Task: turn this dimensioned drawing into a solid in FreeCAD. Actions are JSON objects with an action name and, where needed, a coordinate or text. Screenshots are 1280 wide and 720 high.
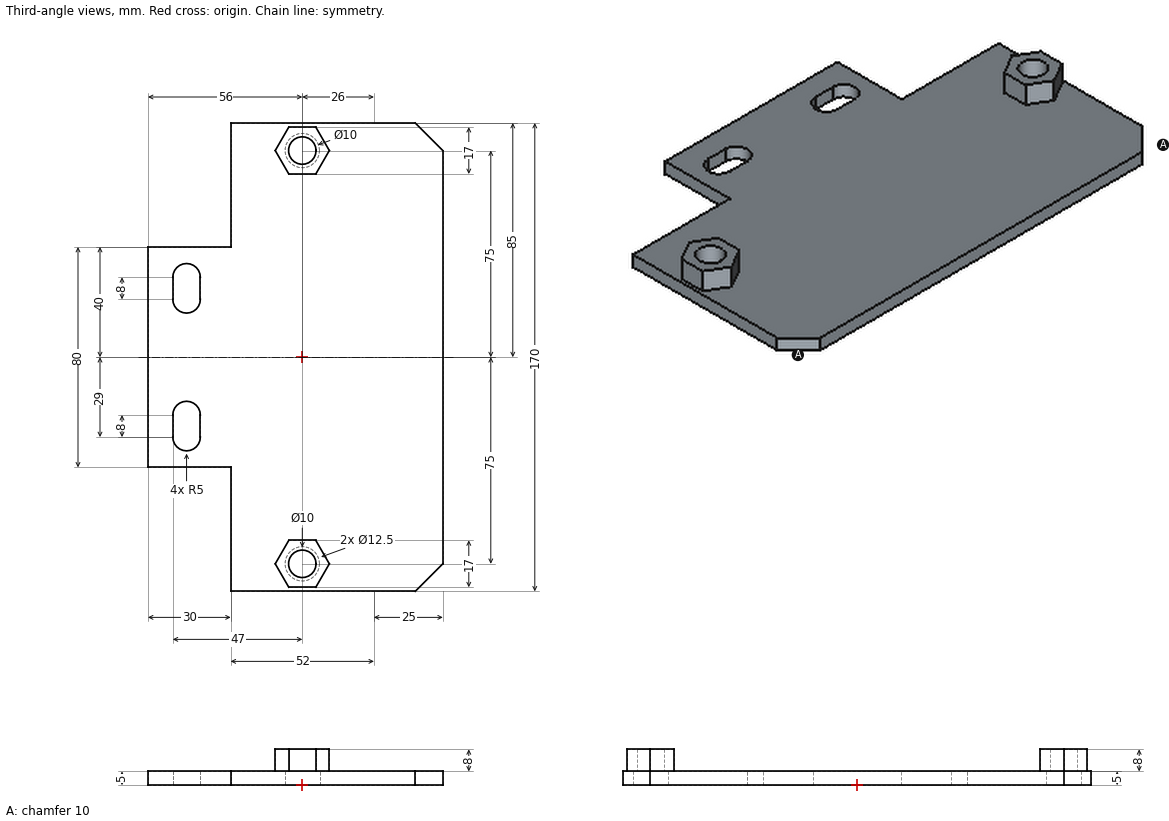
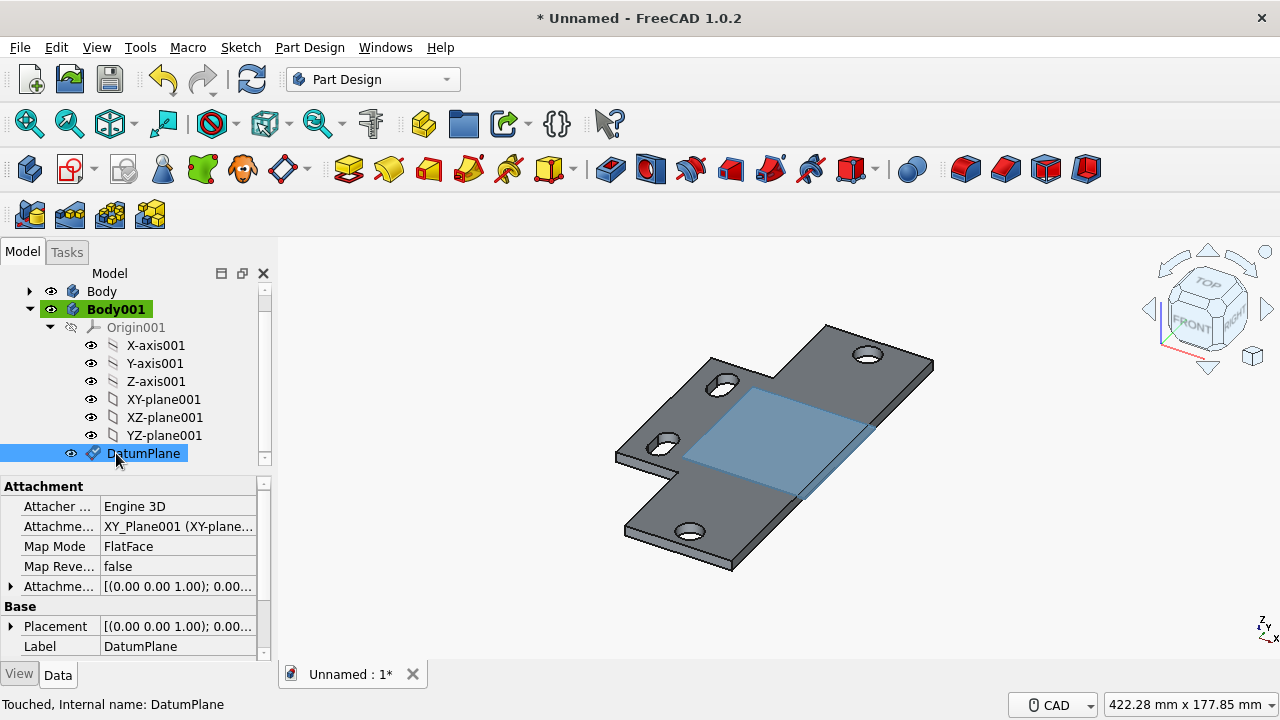
{"action": "left_click", "coordinate": [70, 170]}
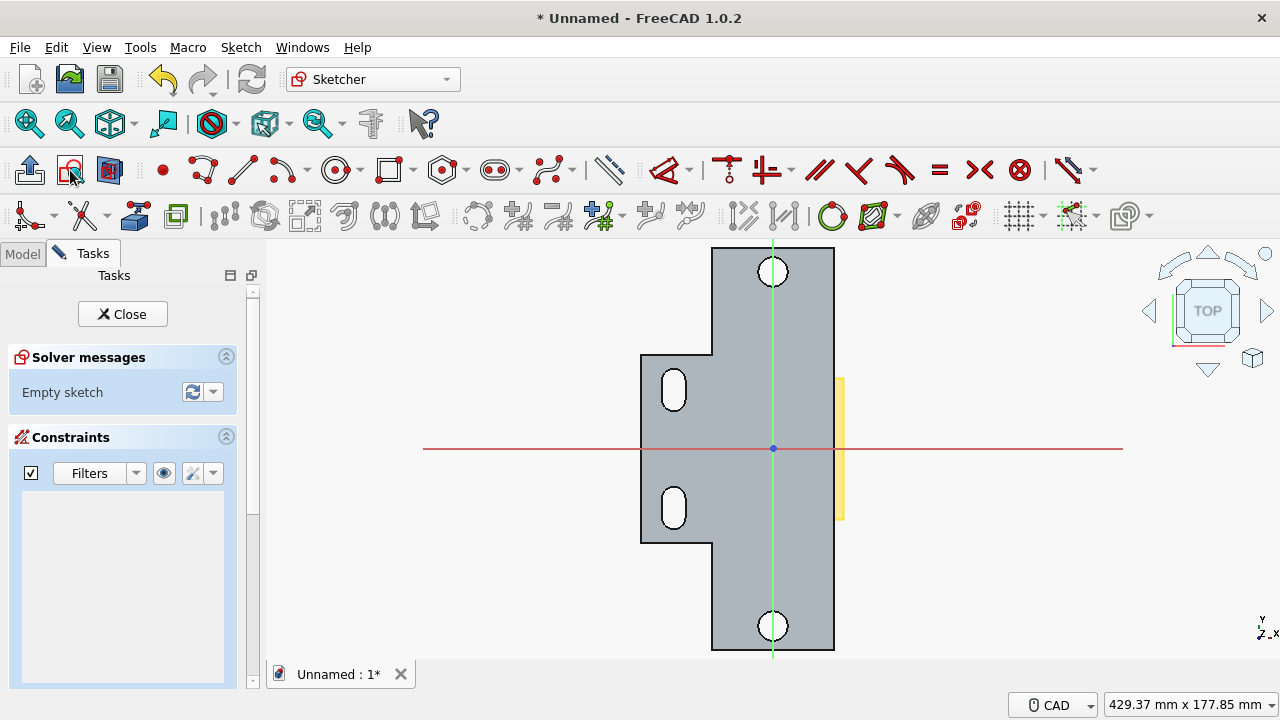
{"action": "scroll", "coordinate": [704, 449], "scroll_direction": "down", "scroll_amount": 5}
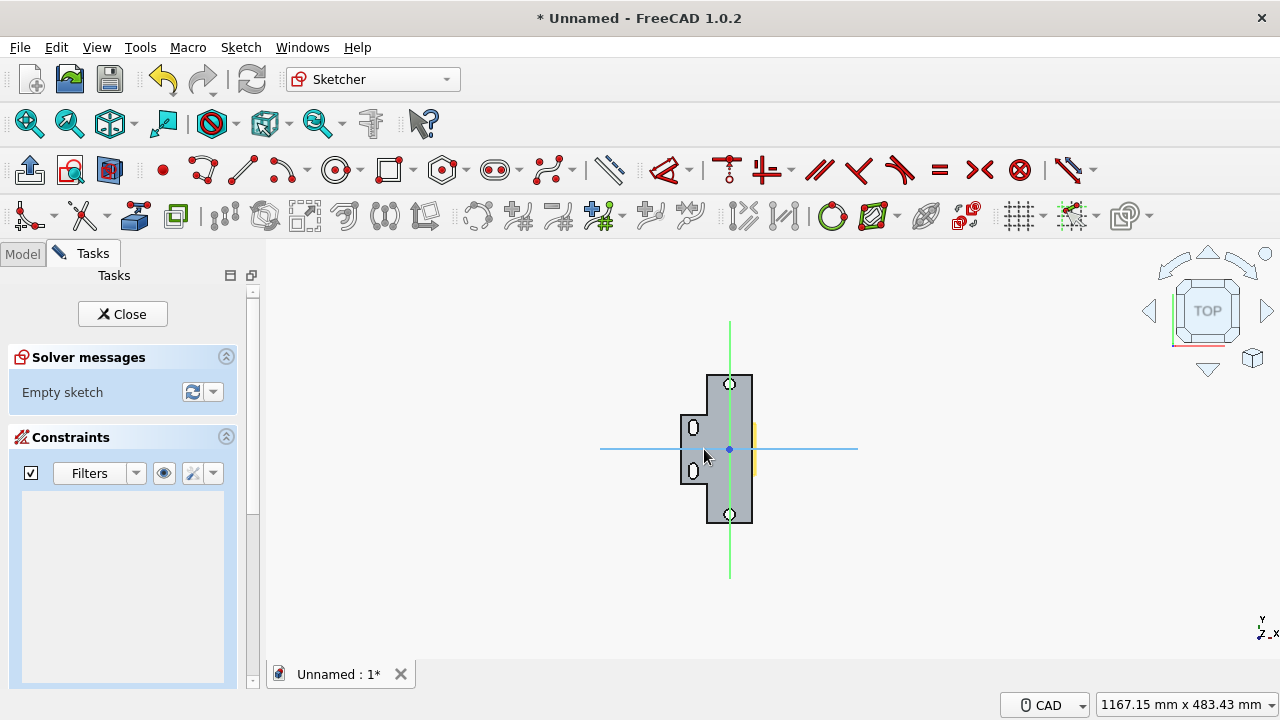
{"action": "scroll", "coordinate": [731, 380], "scroll_direction": "up", "scroll_amount": 14}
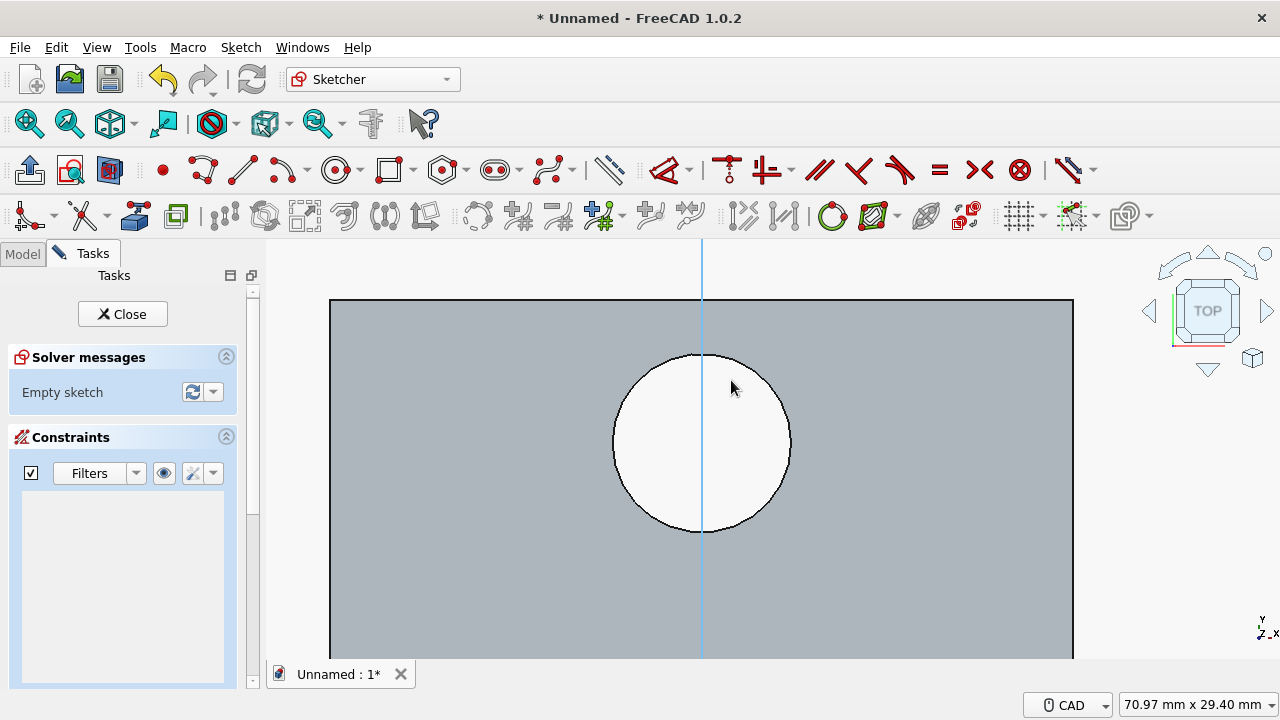
{"action": "left_click", "coordinate": [442, 170]}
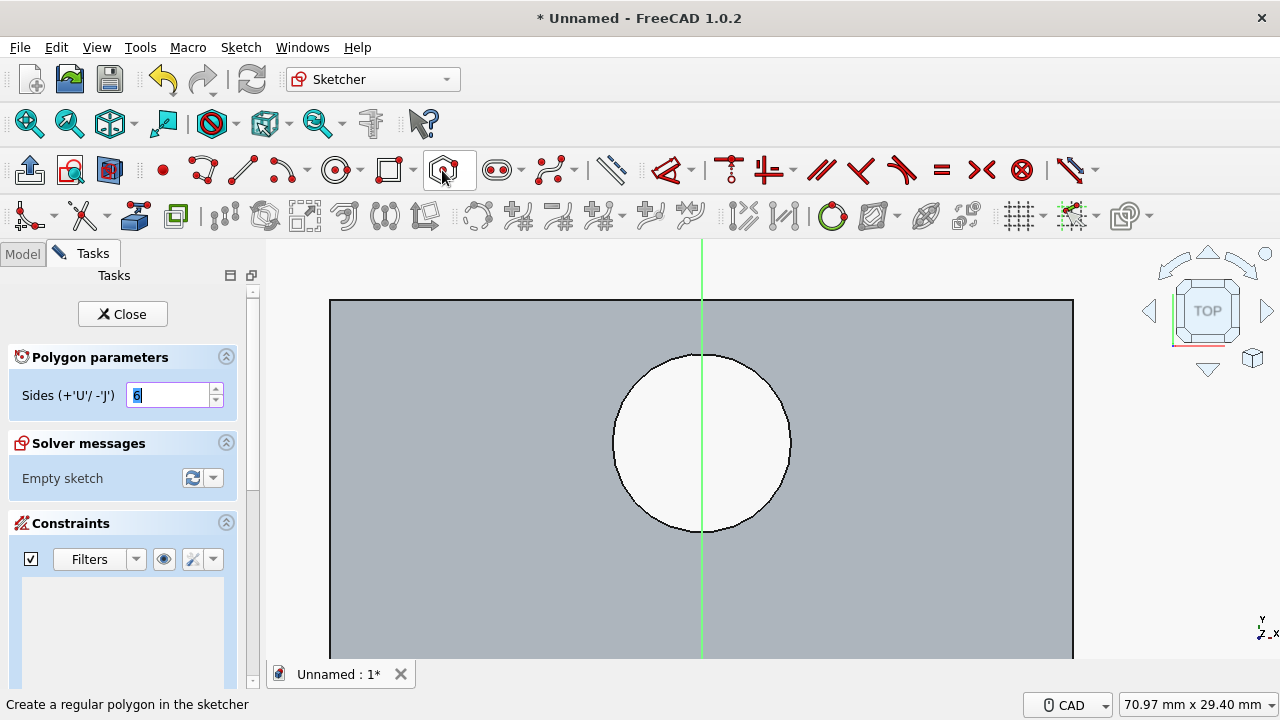
{"action": "left_click", "coordinate": [702, 443]}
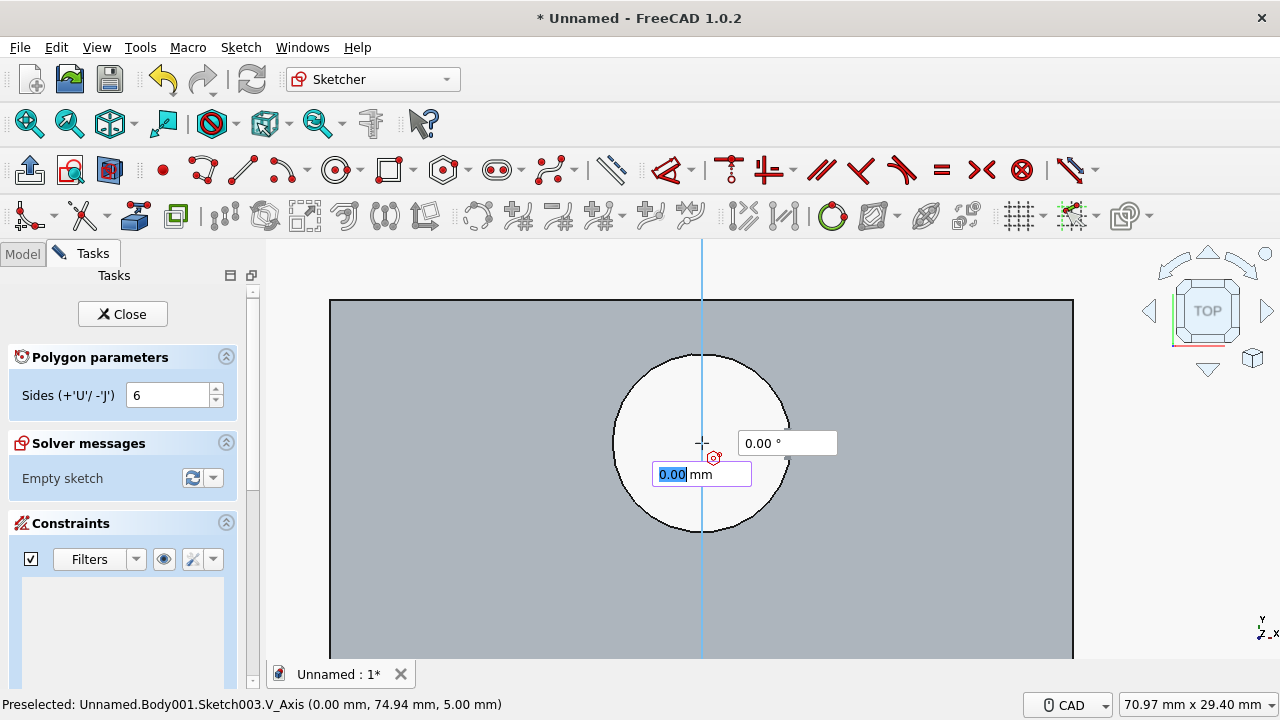
{"action": "left_click", "coordinate": [842, 443]}
{"action": "key", "text": "Escape"}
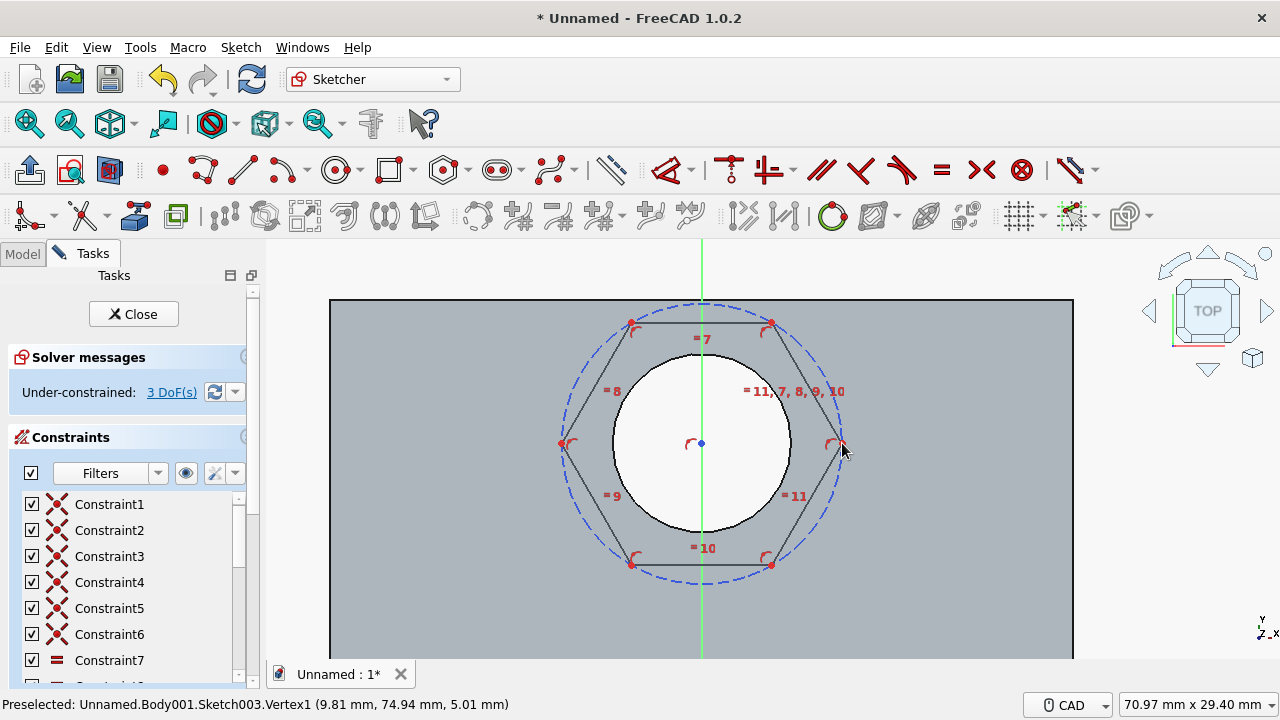
{"action": "left_click", "coordinate": [336, 170]}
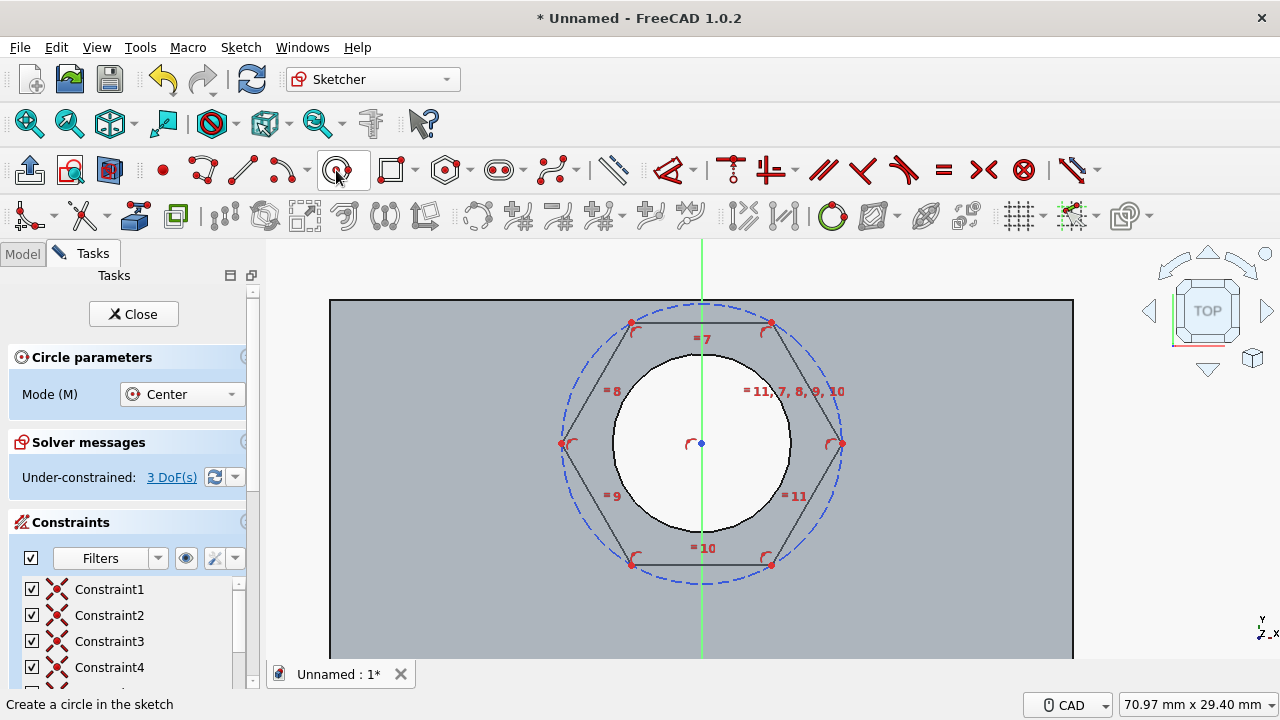
{"action": "left_click", "coordinate": [702, 444]}
{"action": "left_click", "coordinate": [752, 393]}
{"action": "key", "text": "Escape"}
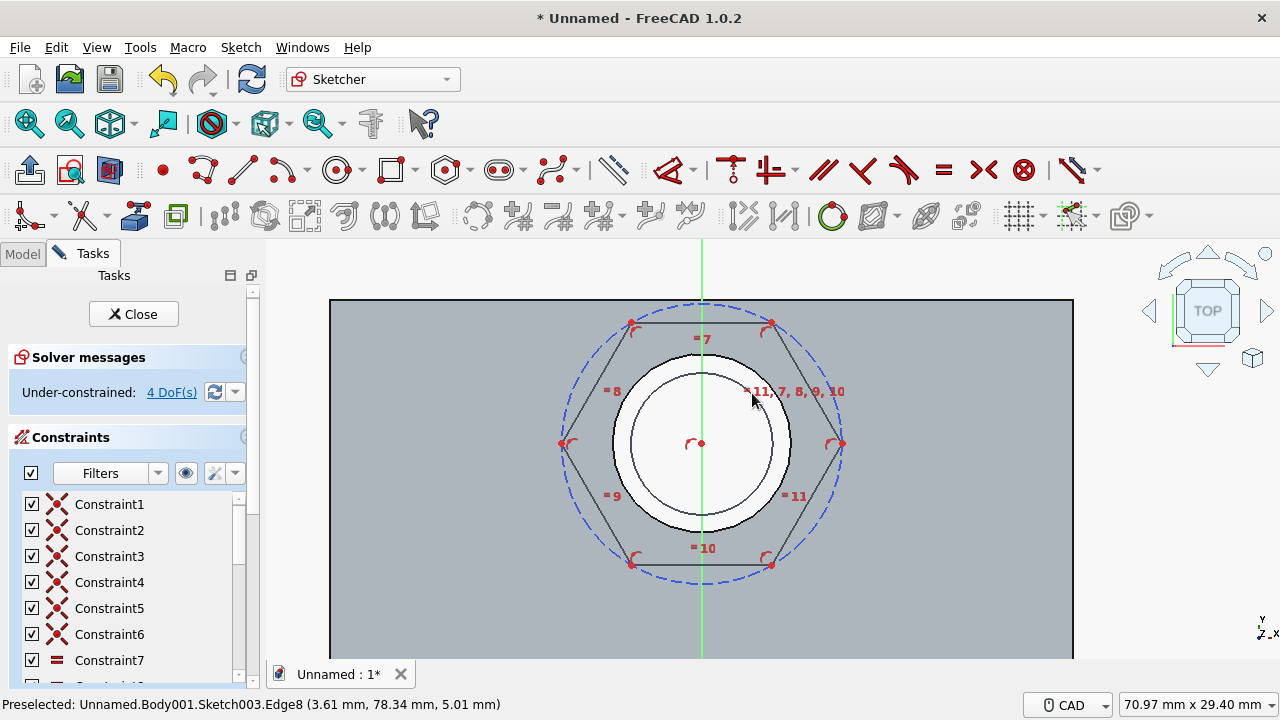
{"action": "left_click", "coordinate": [730, 323]}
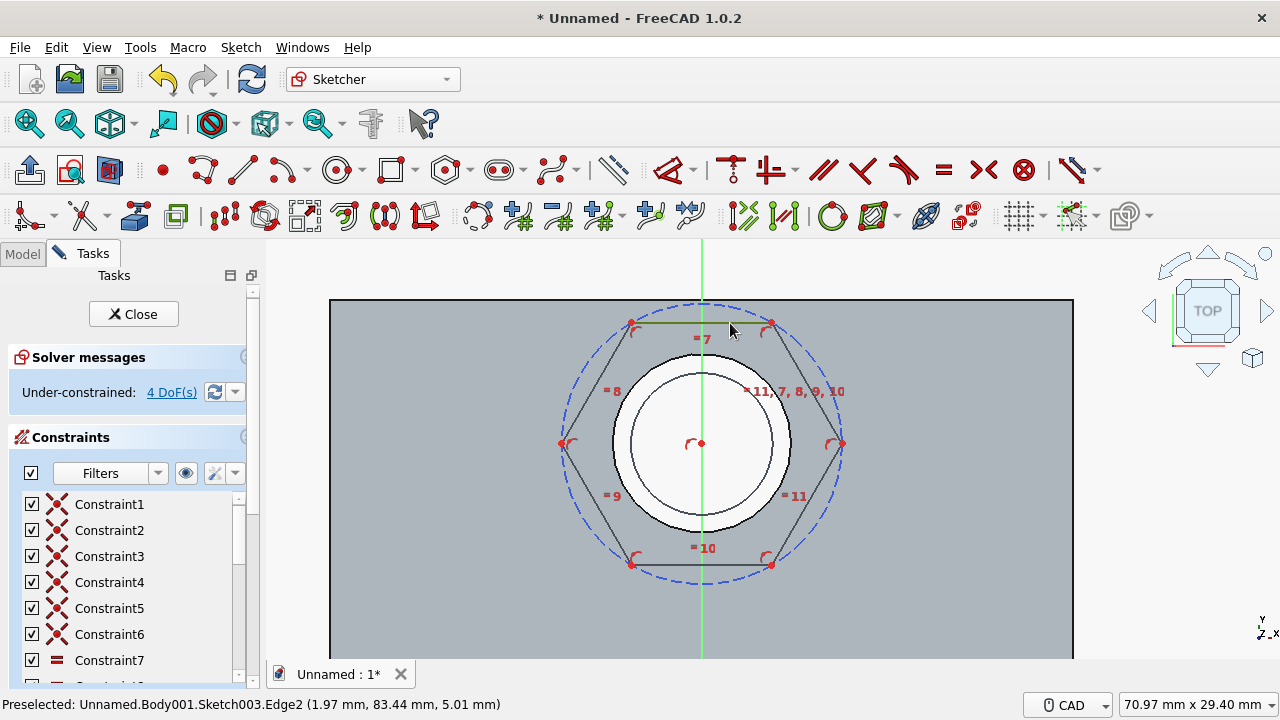
{"action": "left_click", "coordinate": [798, 170]}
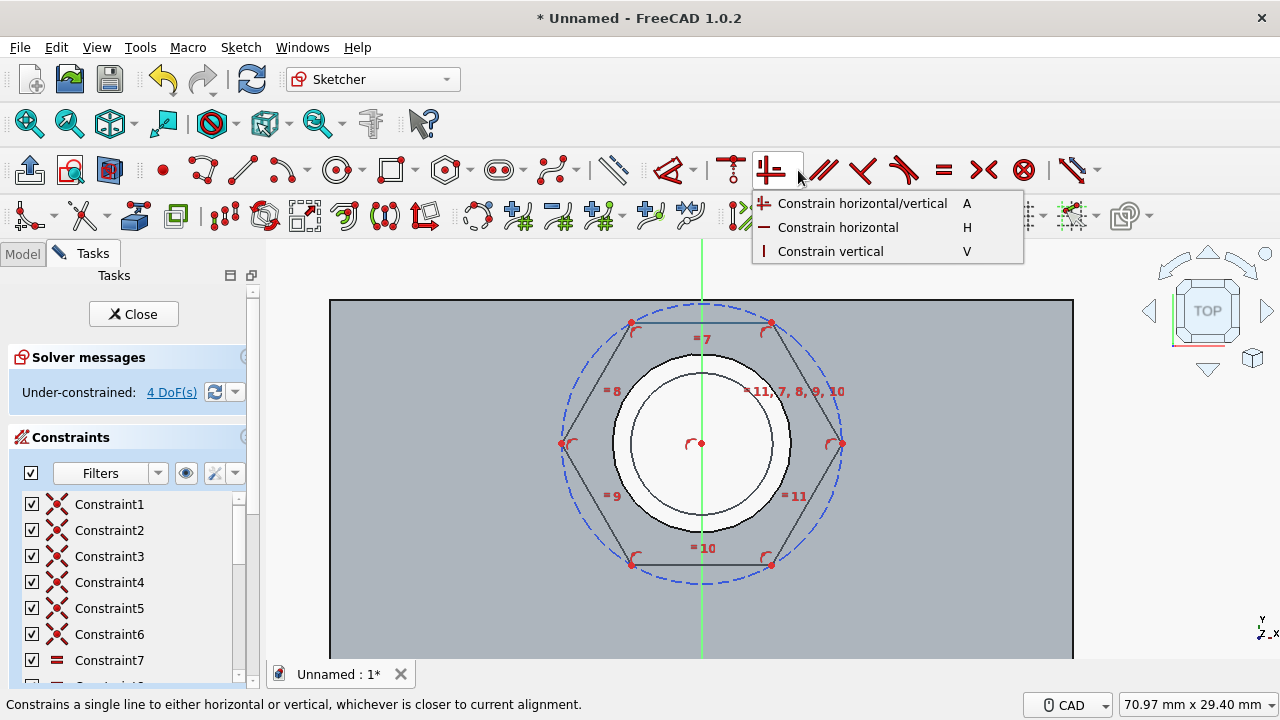
{"action": "left_click", "coordinate": [888, 227]}